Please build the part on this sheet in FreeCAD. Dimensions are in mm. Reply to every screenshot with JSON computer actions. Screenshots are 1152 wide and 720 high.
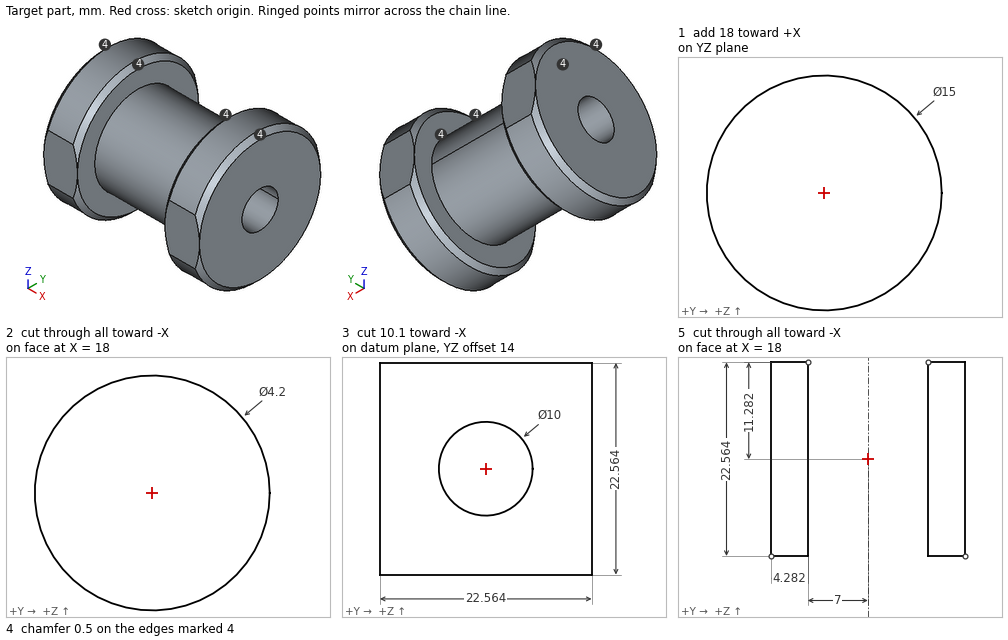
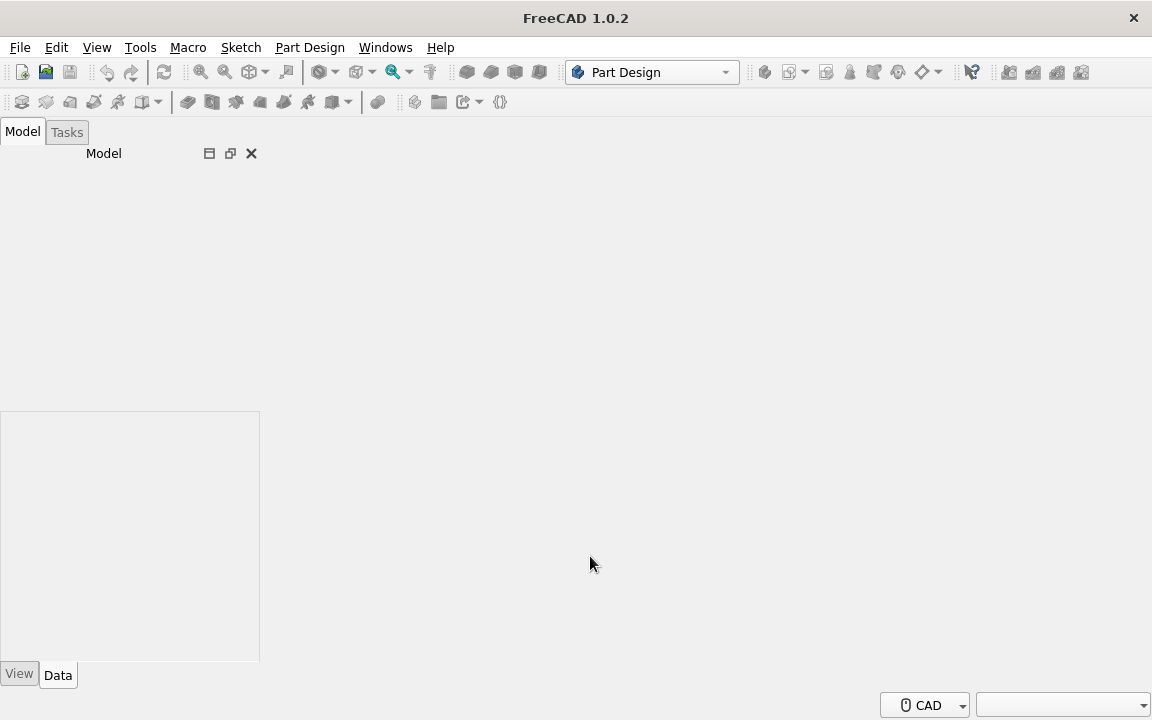
{"action": "left_click", "coordinate": [22, 72]}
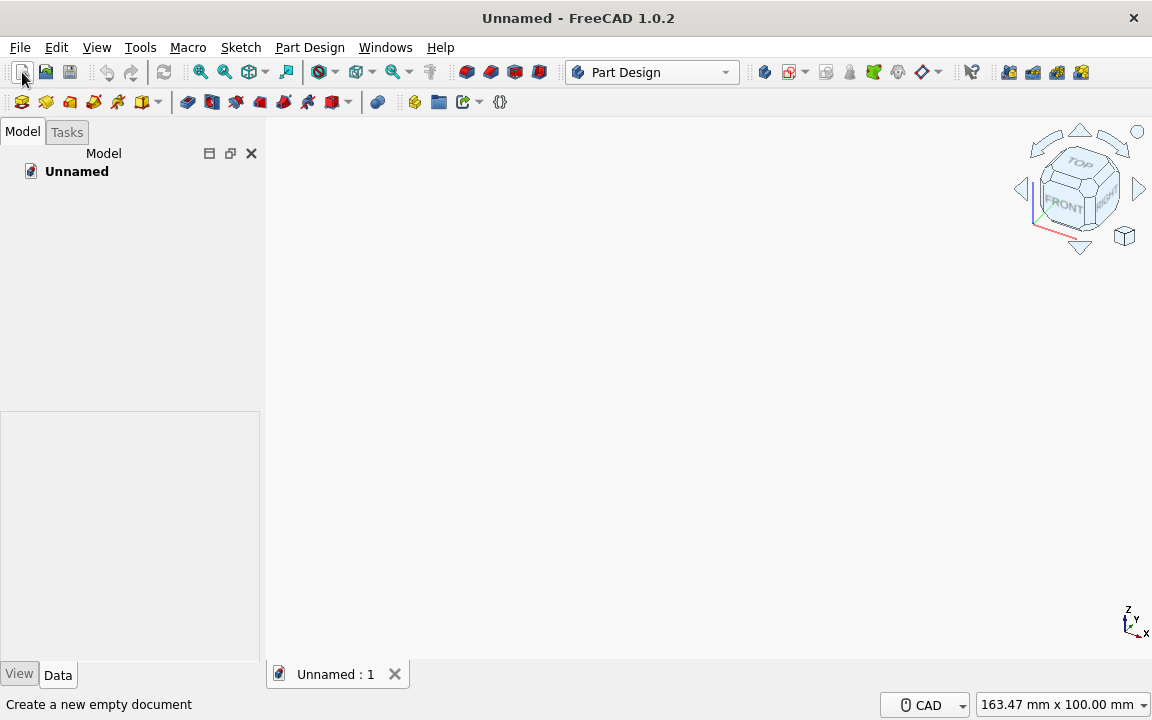
{"action": "left_click", "coordinate": [790, 72]}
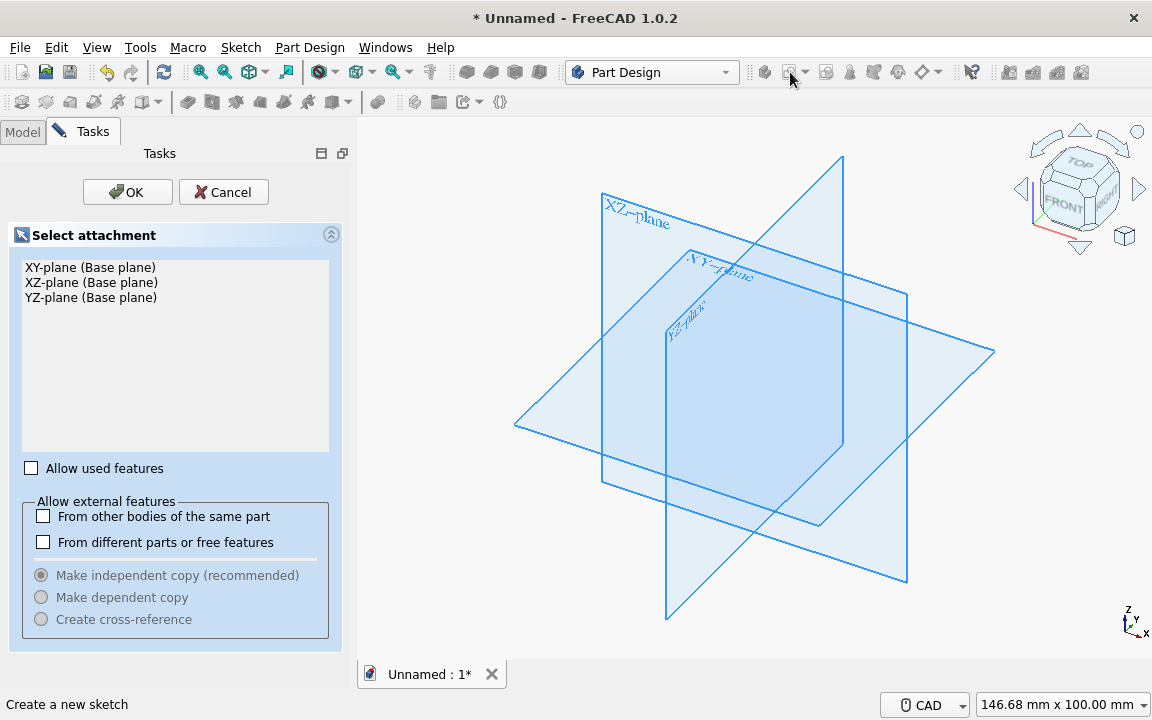
{"action": "left_click", "coordinate": [82, 298]}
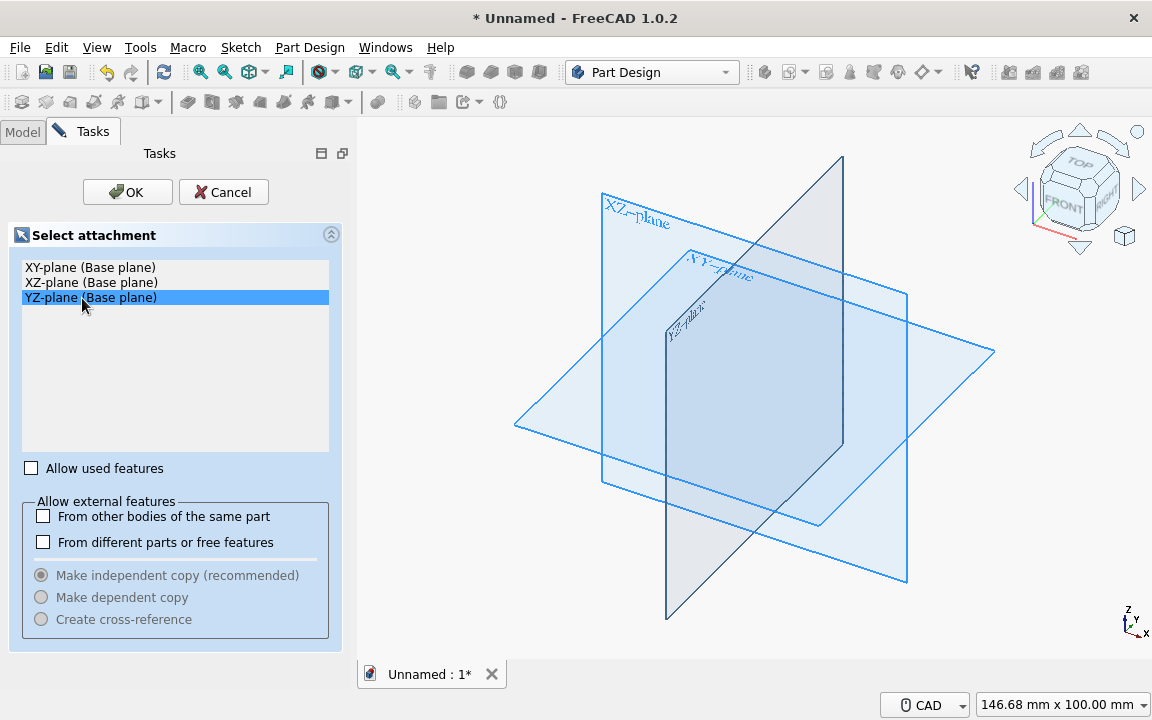
{"action": "left_click", "coordinate": [128, 192]}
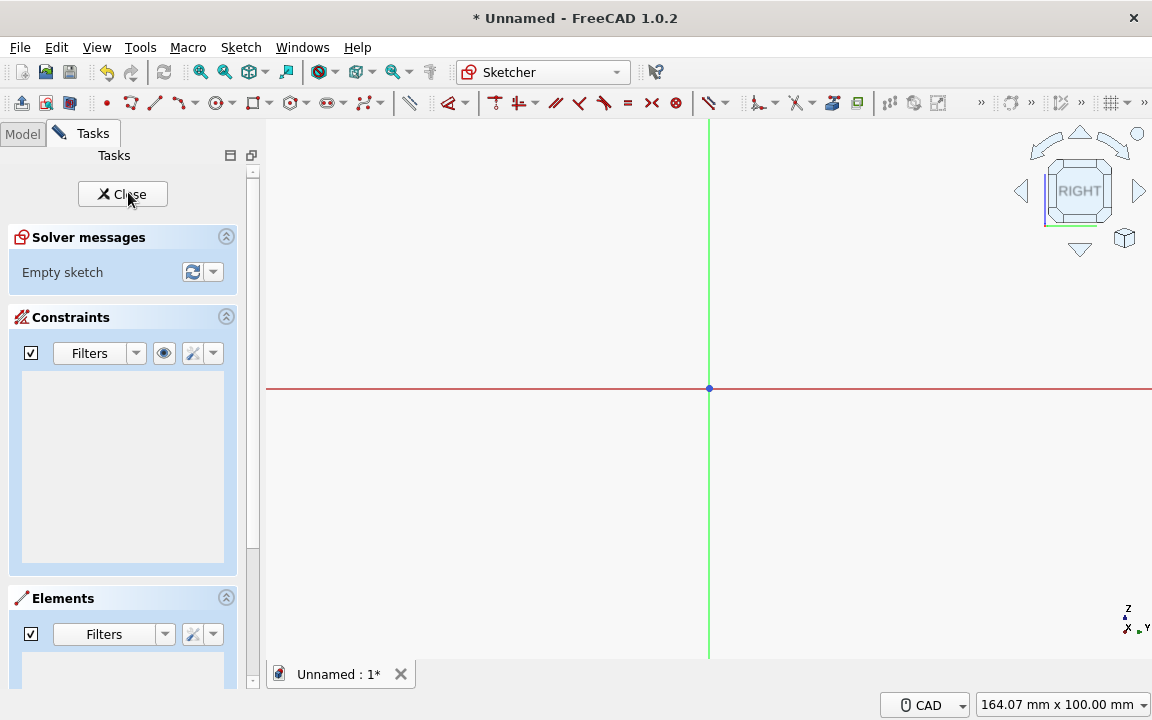
{"action": "scroll", "coordinate": [731, 389], "scroll_direction": "up", "scroll_amount": 7}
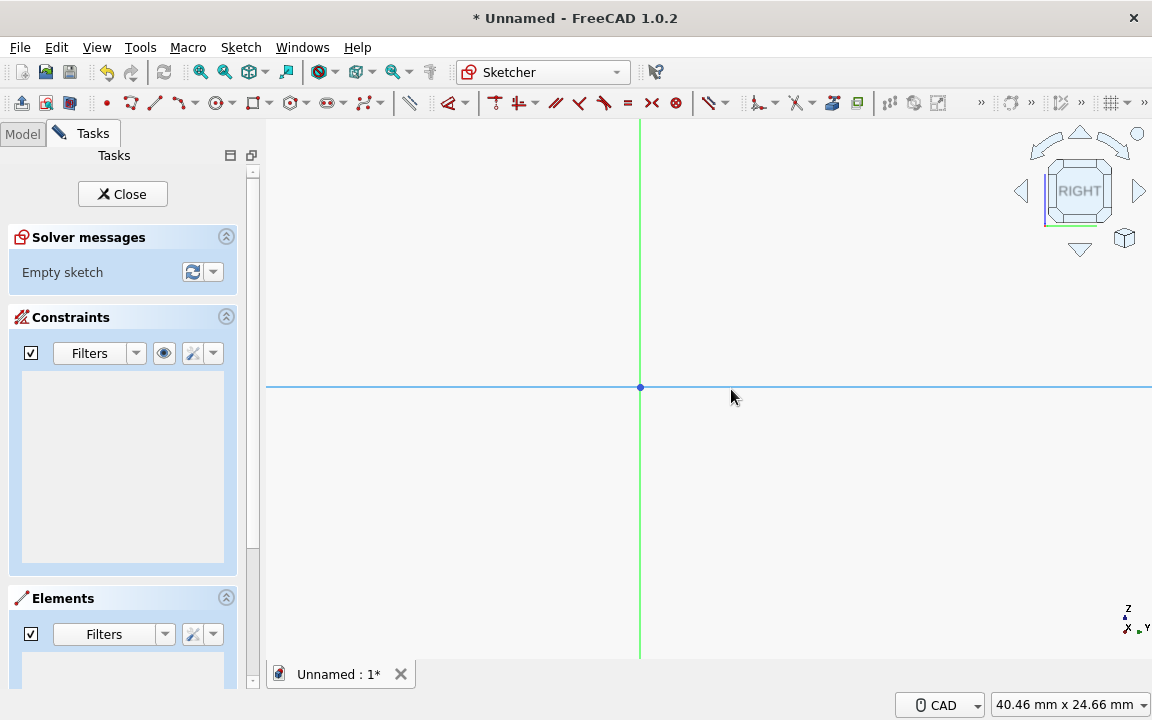
{"action": "left_click", "coordinate": [216, 104]}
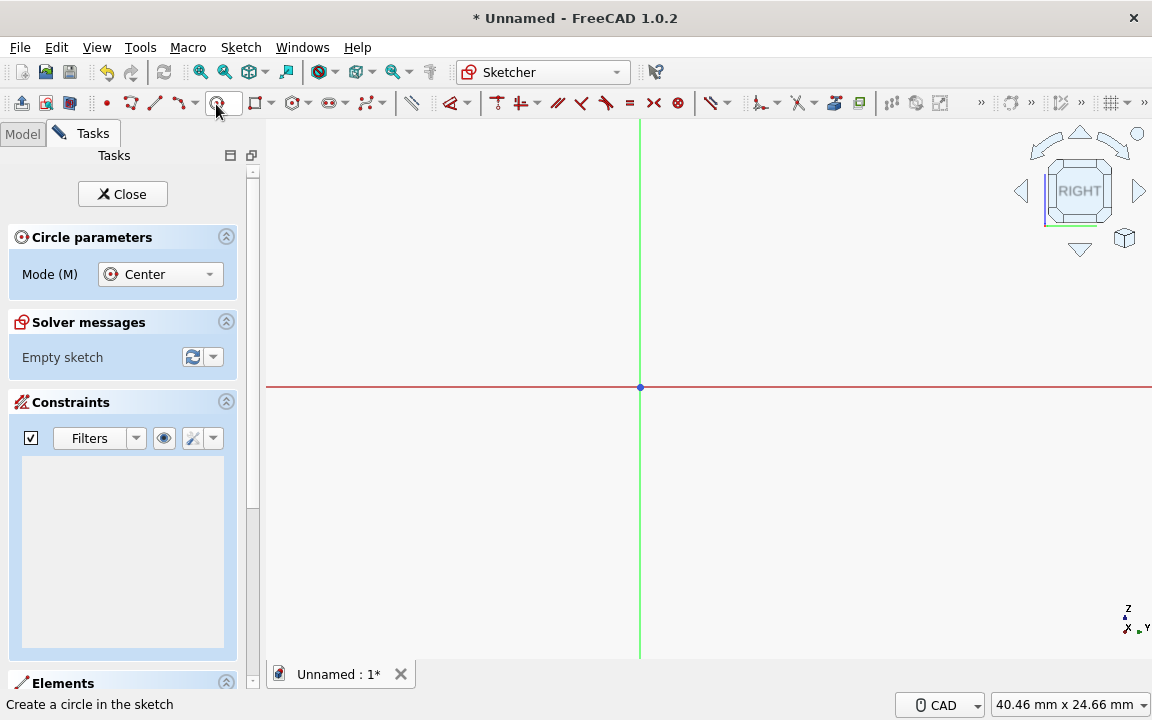
{"action": "left_click", "coordinate": [640, 387]}
{"action": "left_click", "coordinate": [756, 271]}
{"action": "key", "text": "Escape"}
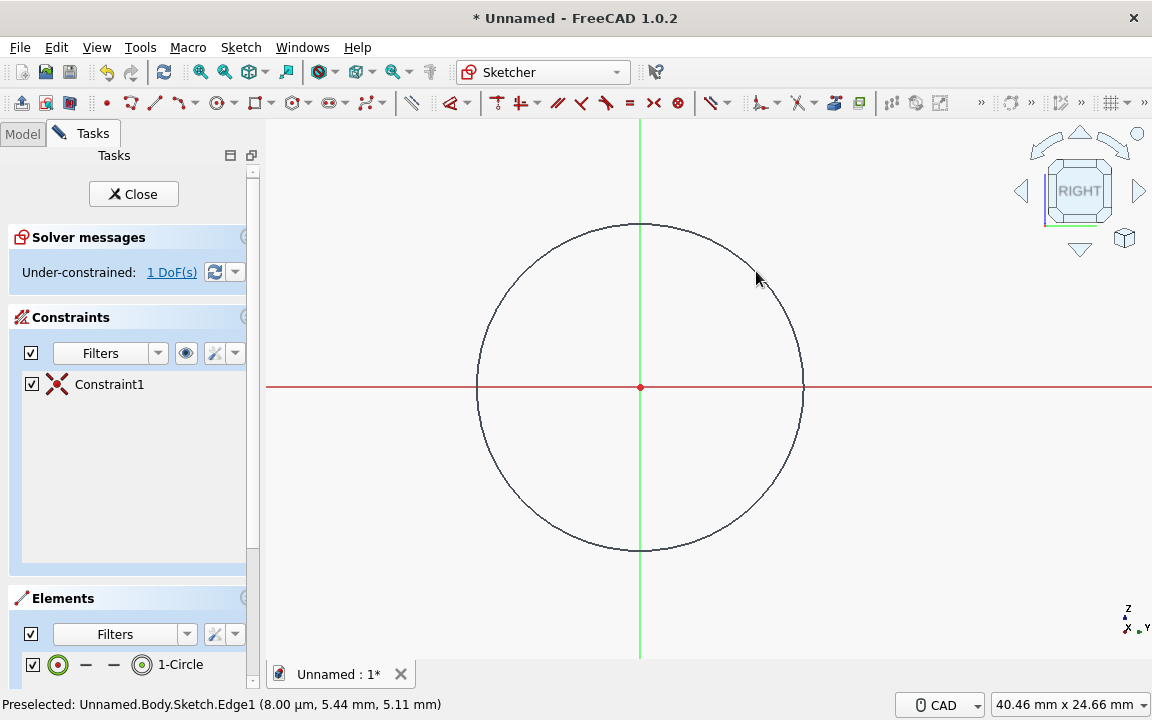
{"action": "left_click", "coordinate": [450, 104]}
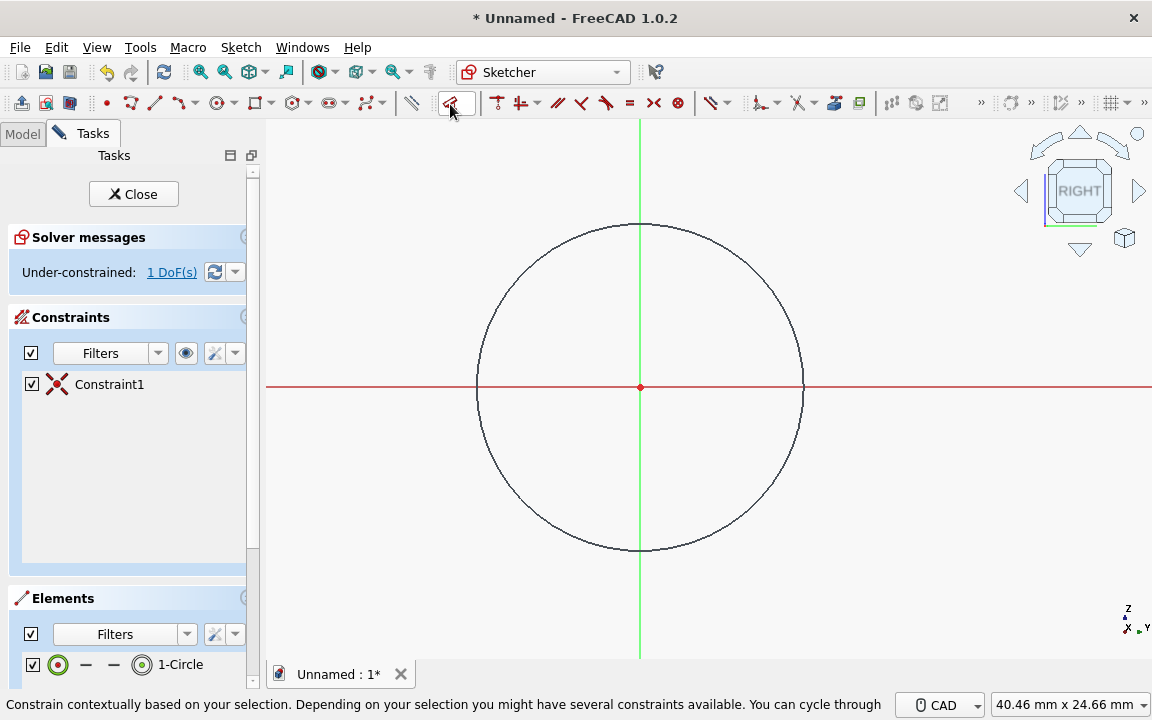
{"action": "left_click", "coordinate": [755, 271]}
{"action": "left_click", "coordinate": [777, 248]}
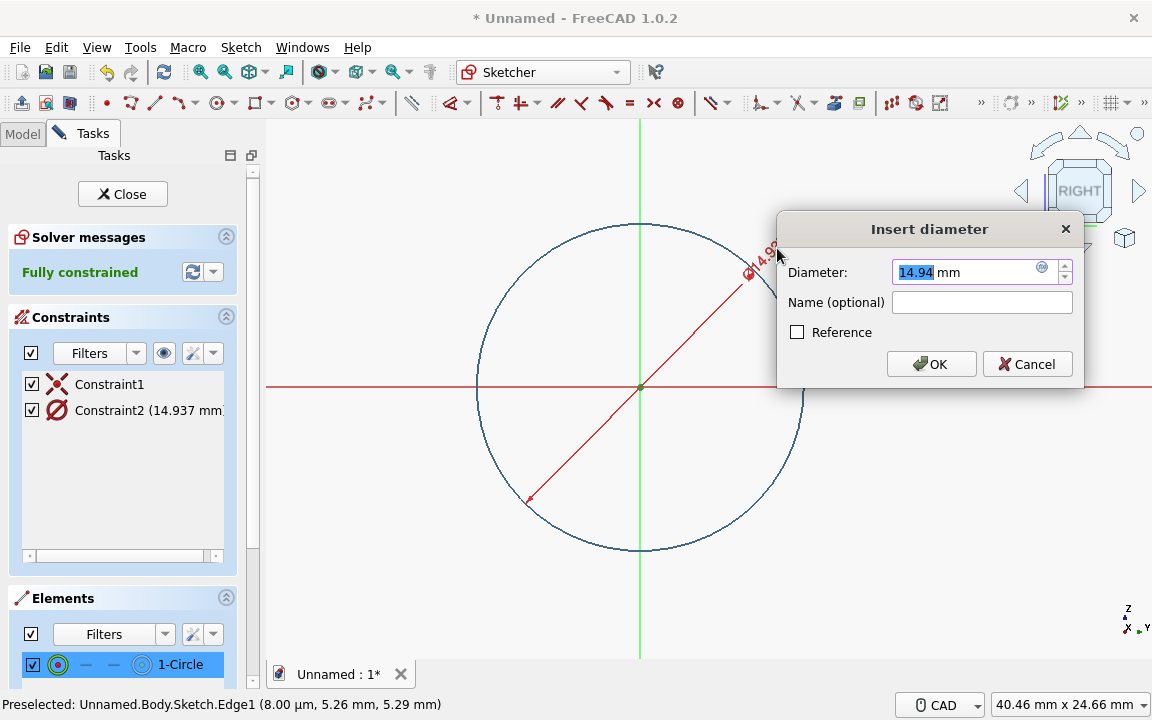
{"action": "type", "text": "15"}
{"action": "key", "text": "Return"}
{"action": "key", "text": "Escape"}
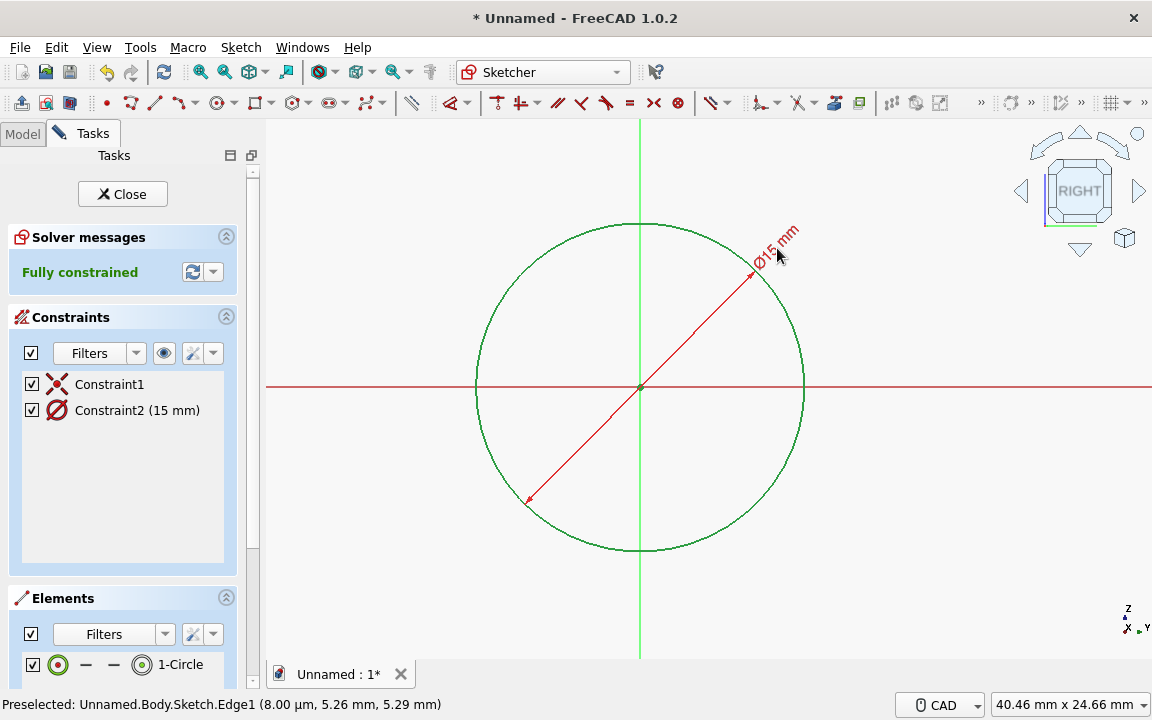
{"action": "left_click", "coordinate": [123, 194]}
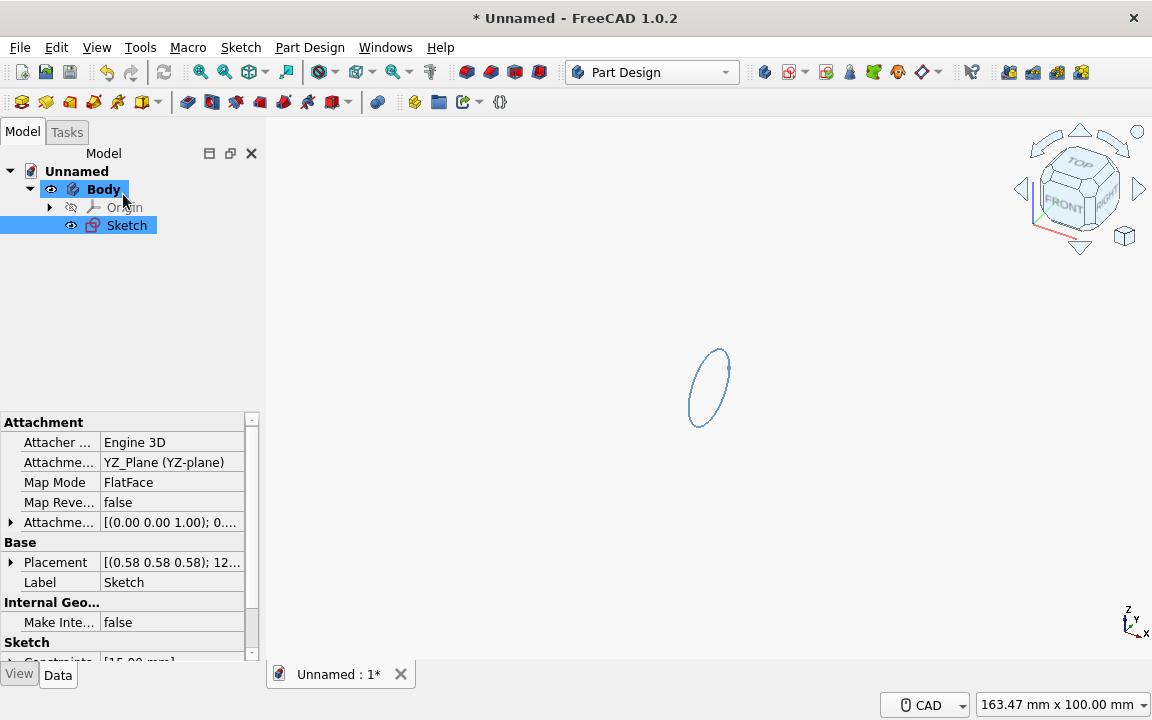
{"action": "left_click", "coordinate": [22, 102]}